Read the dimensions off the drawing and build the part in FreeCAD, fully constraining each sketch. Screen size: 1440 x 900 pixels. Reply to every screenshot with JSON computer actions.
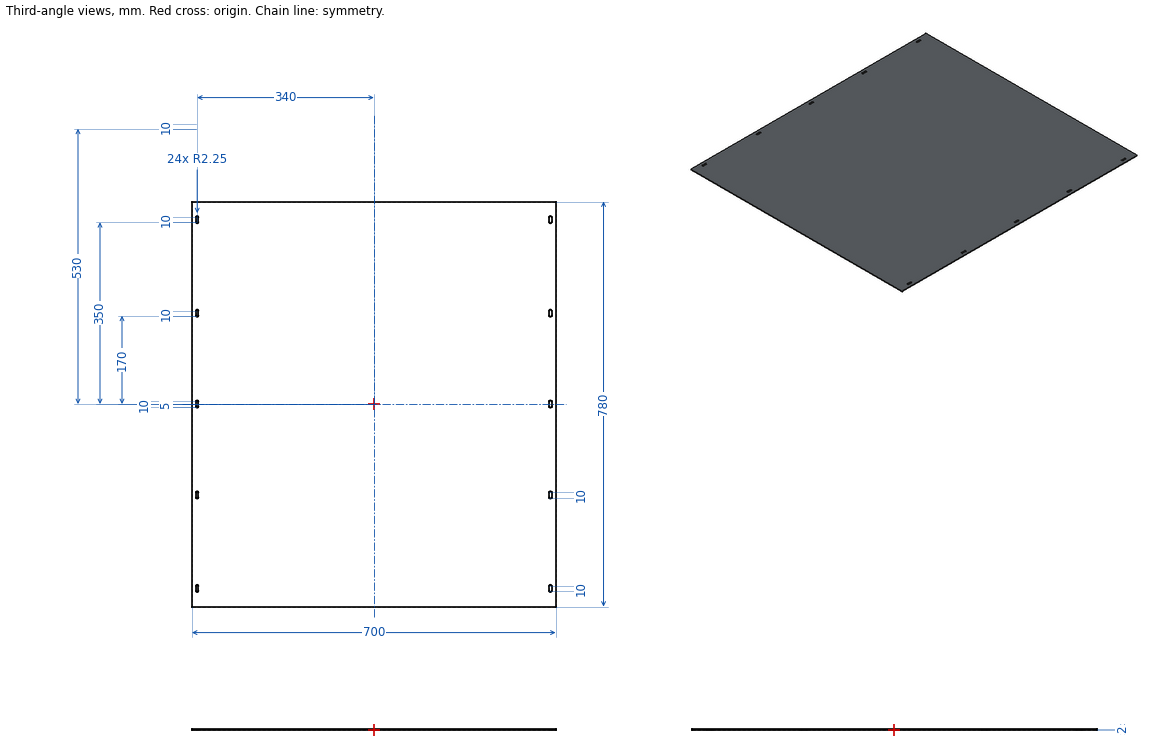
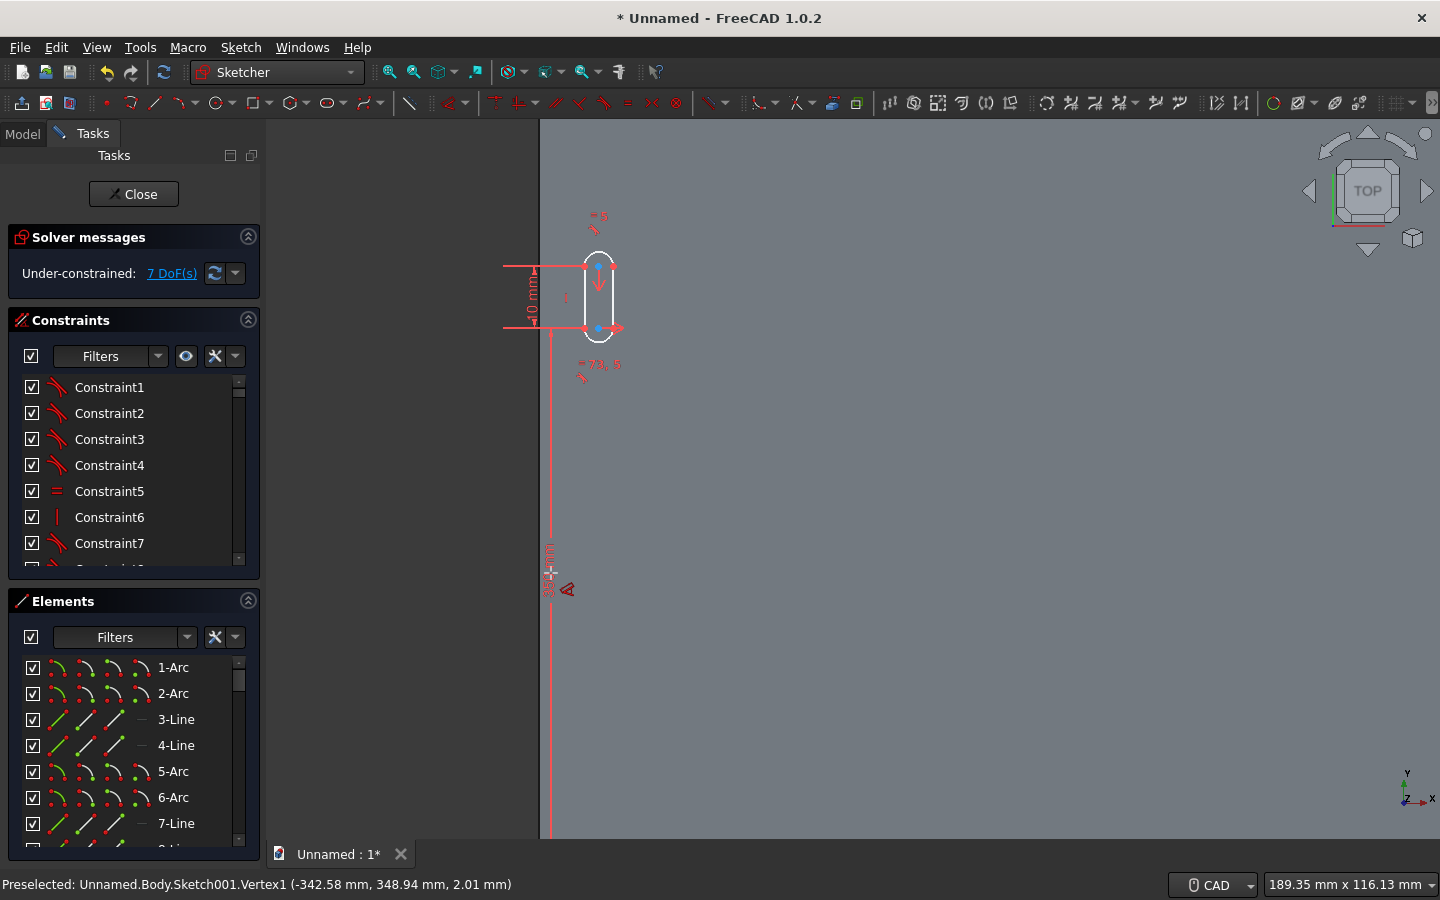
{"action": "scroll", "coordinate": [593, 333], "scroll_direction": "down", "scroll_amount": 12}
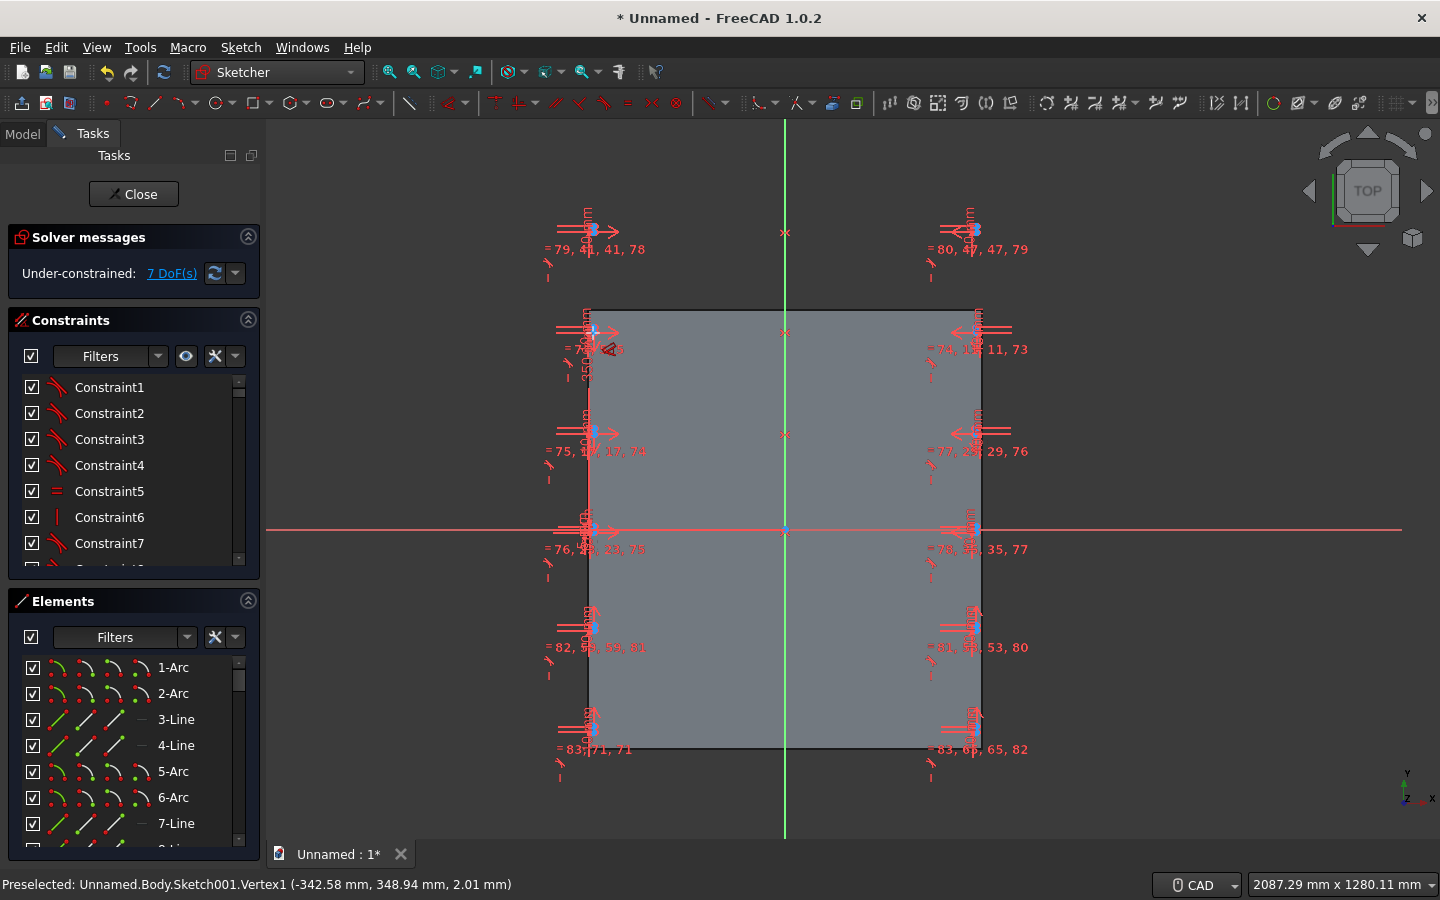
{"action": "scroll", "coordinate": [593, 434], "scroll_direction": "up", "scroll_amount": 12}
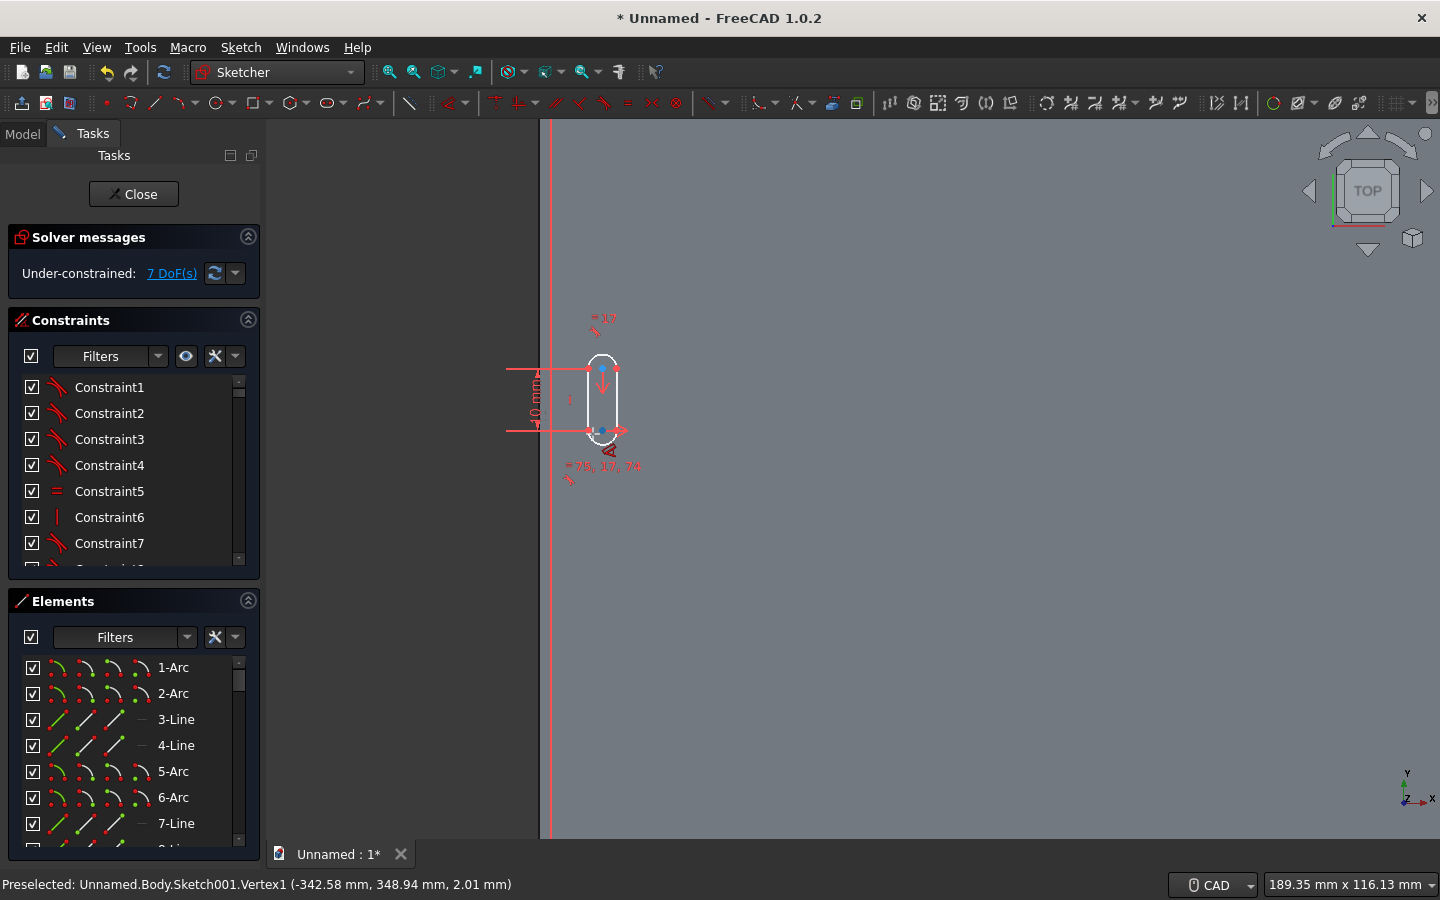
{"action": "left_click", "coordinate": [588, 431]}
{"action": "left_click", "coordinate": [554, 621]}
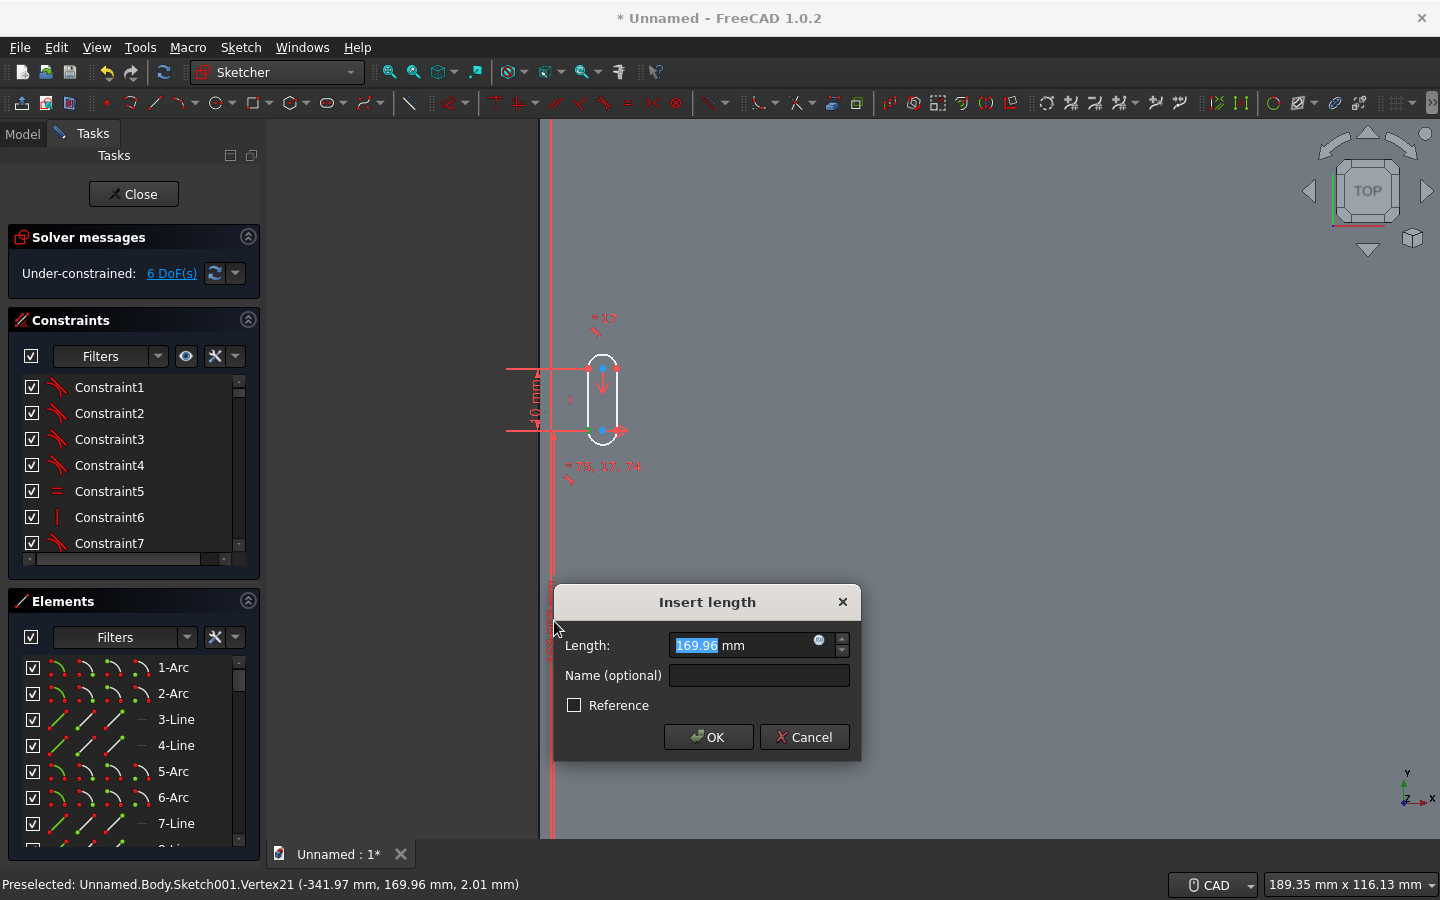
{"action": "type", "text": "170"}
{"action": "key", "text": "Return"}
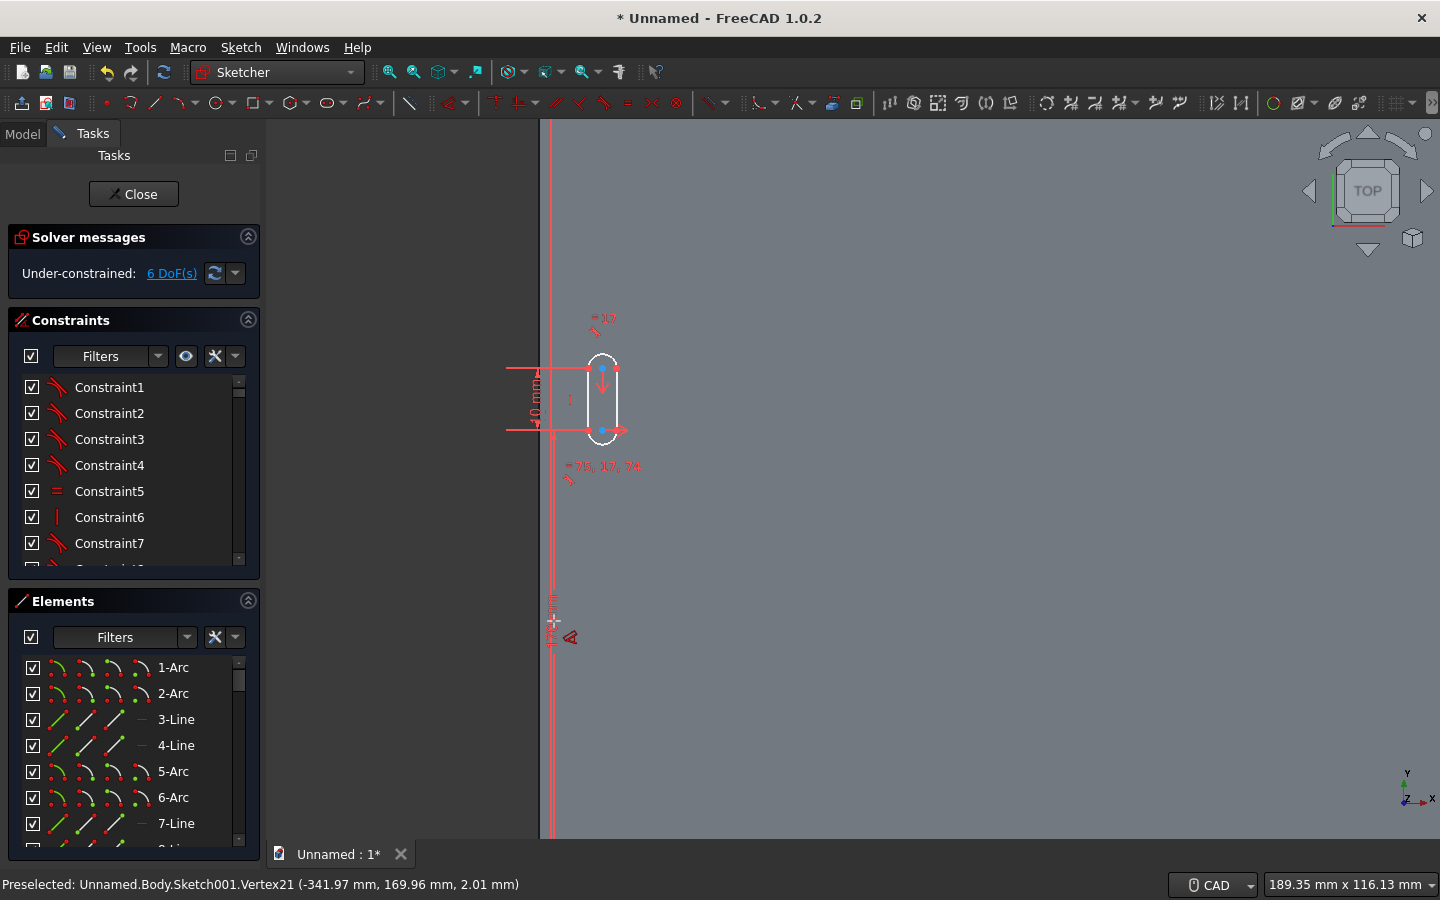
{"action": "scroll", "coordinate": [593, 434], "scroll_direction": "down", "scroll_amount": 12}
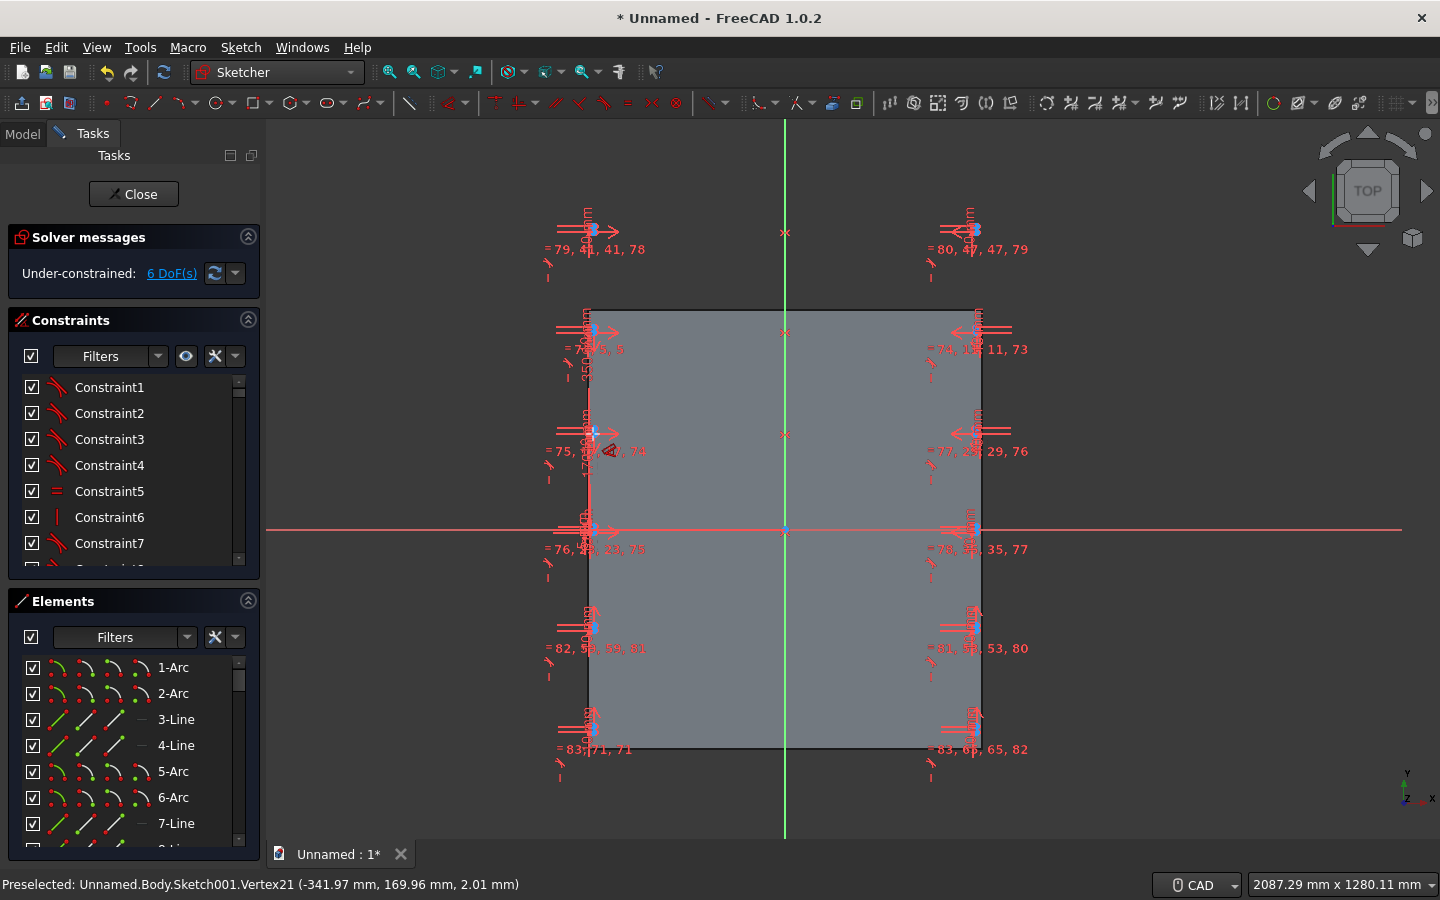
{"action": "scroll", "coordinate": [593, 232], "scroll_direction": "up", "scroll_amount": 12}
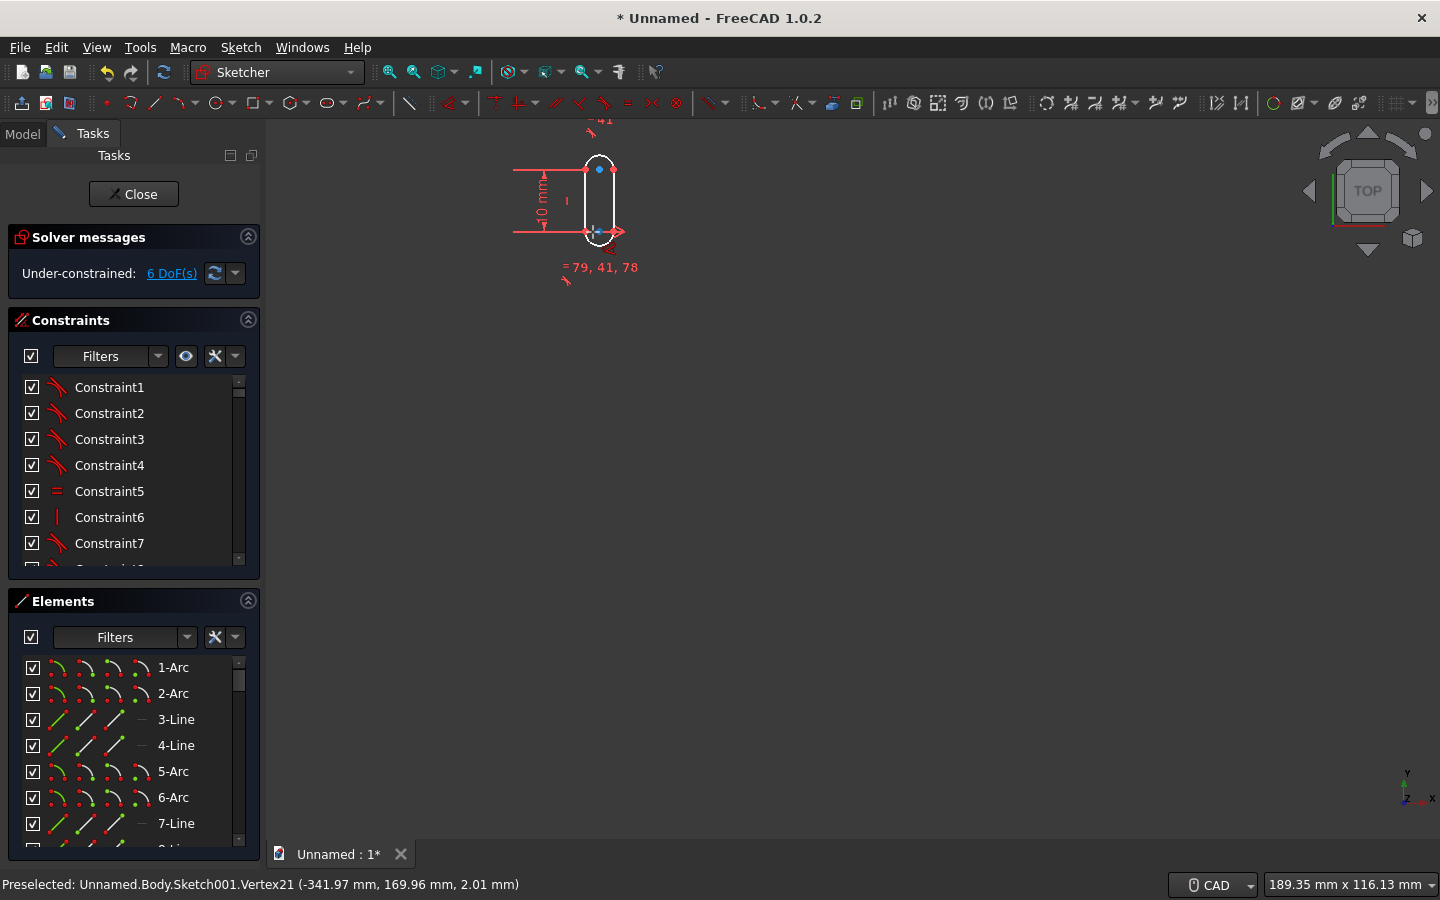
{"action": "left_click", "coordinate": [585, 232]}
{"action": "left_click", "coordinate": [551, 521]}